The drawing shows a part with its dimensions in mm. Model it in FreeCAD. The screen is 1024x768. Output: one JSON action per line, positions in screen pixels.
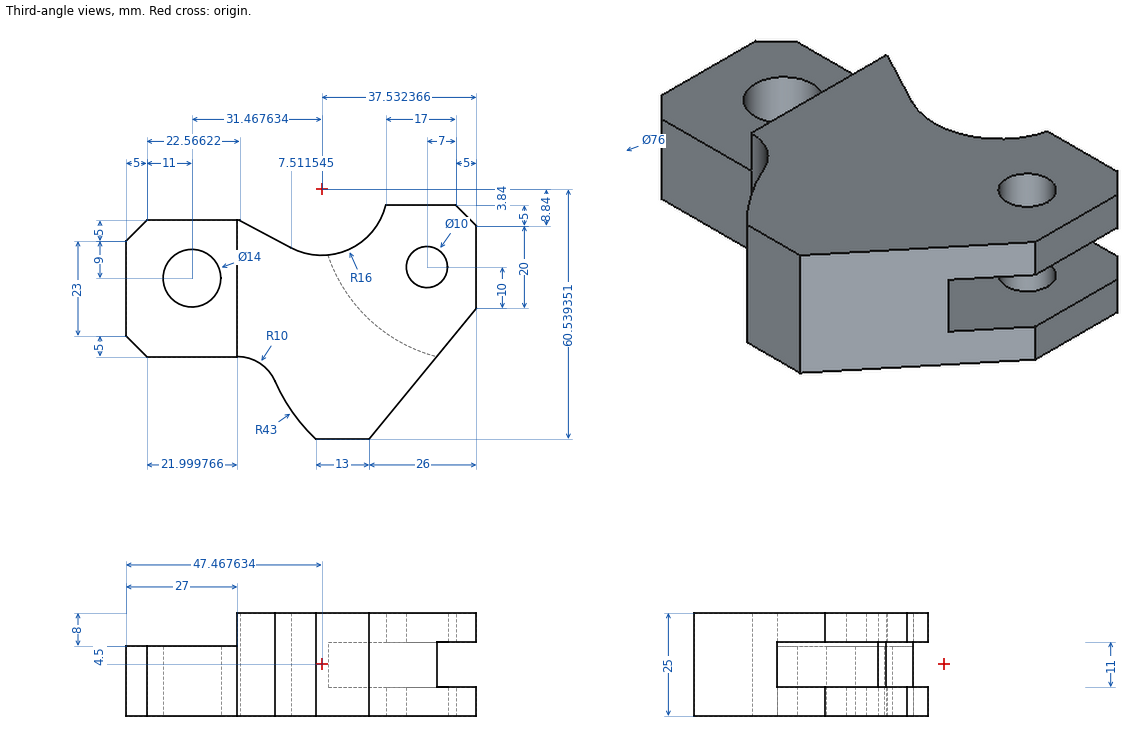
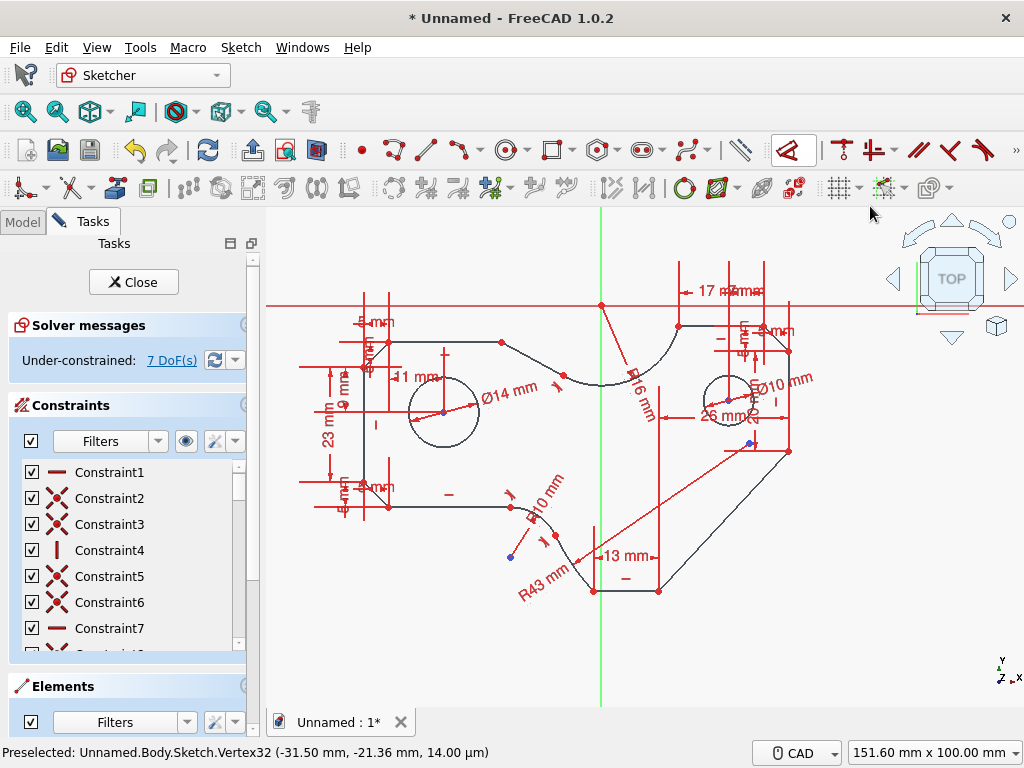
{"action": "left_click", "coordinate": [789, 451]}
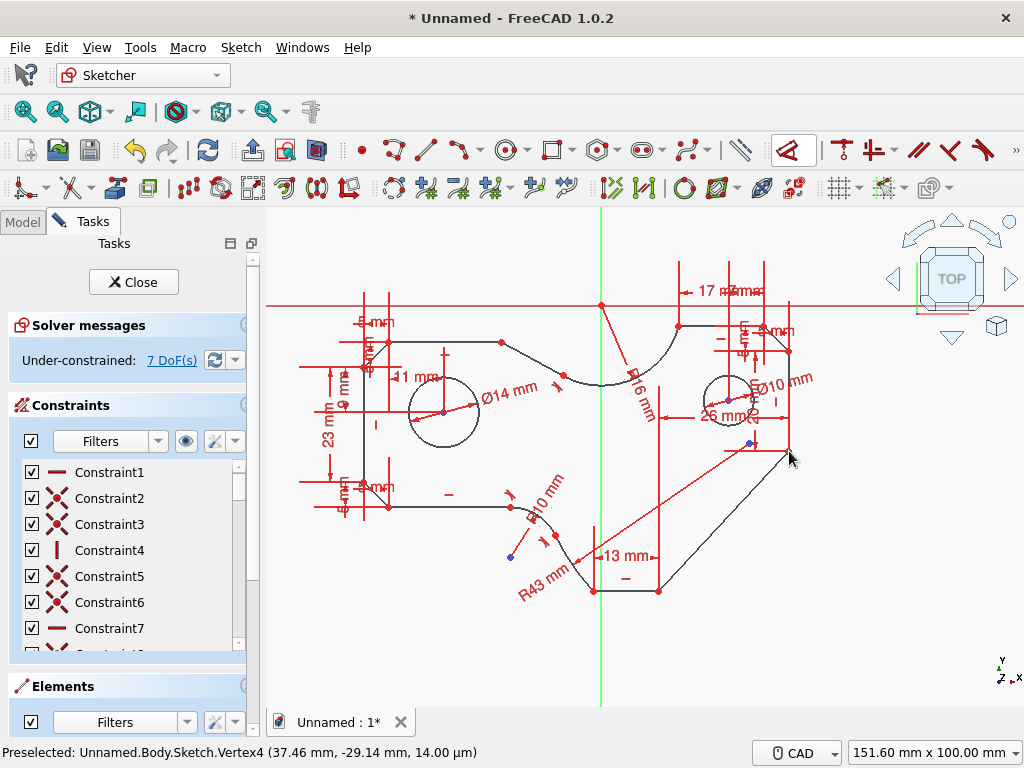
{"action": "left_click", "coordinate": [729, 401]}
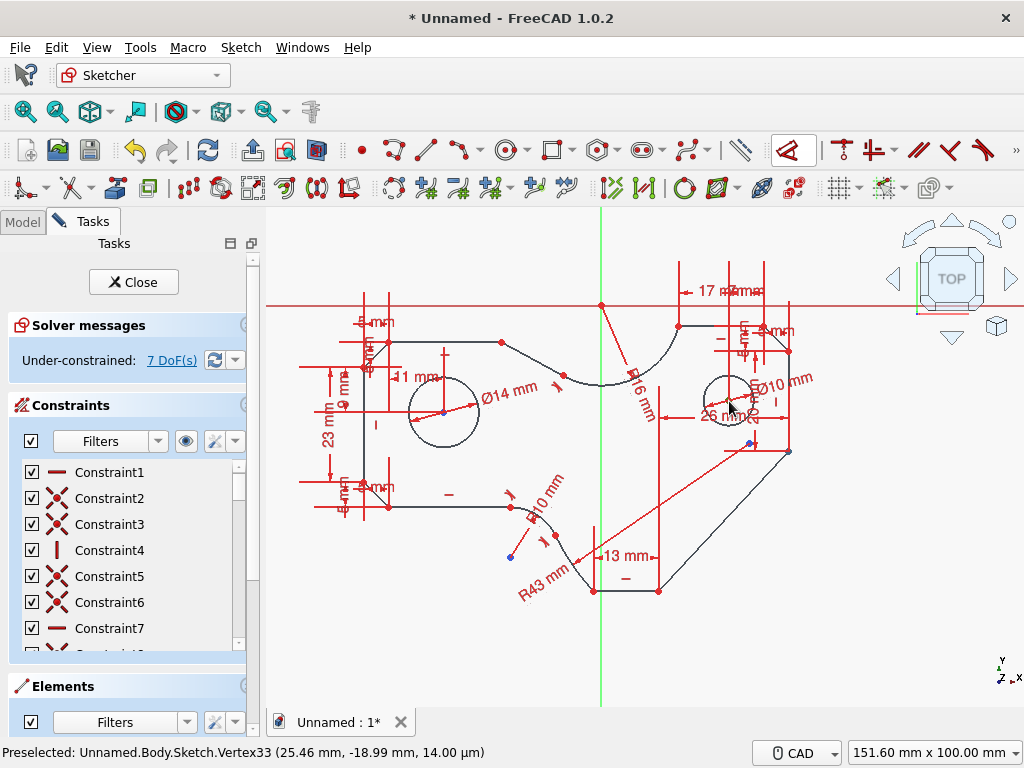
{"action": "left_click", "coordinate": [810, 150]}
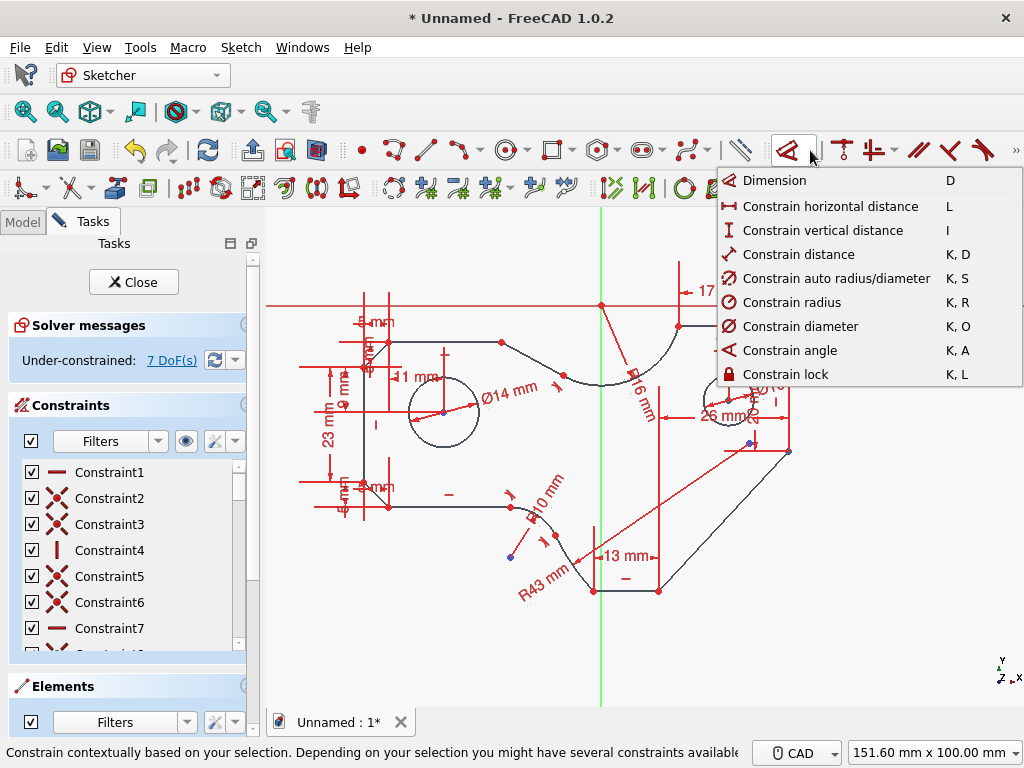
{"action": "left_click", "coordinate": [870, 230]}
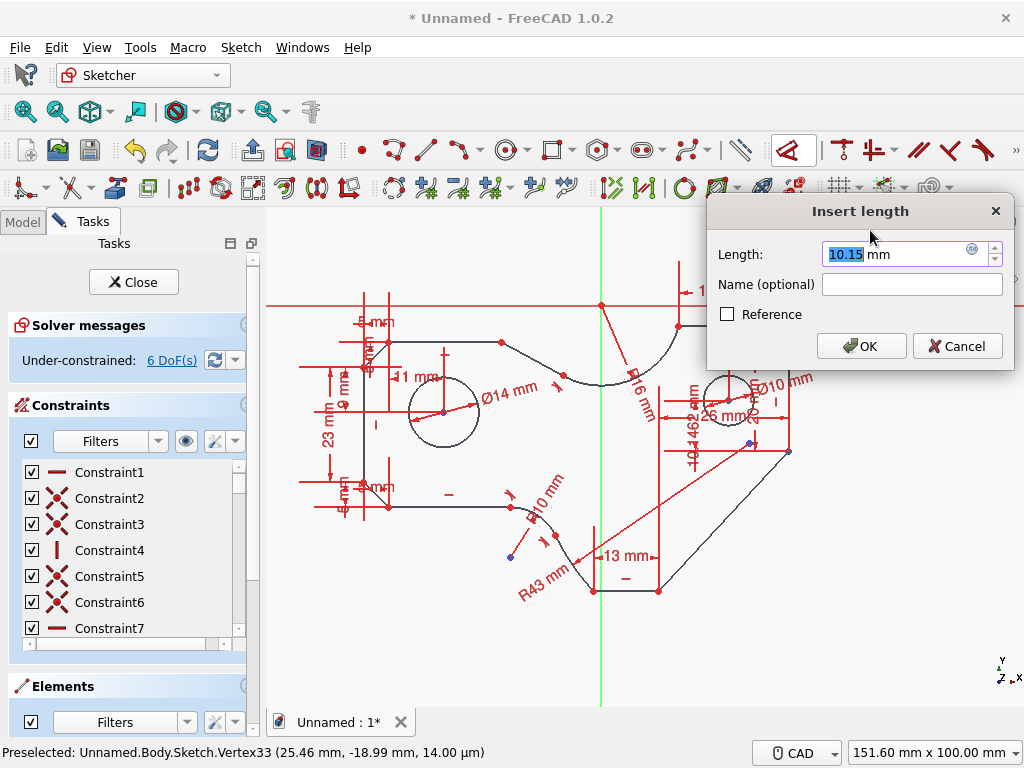
{"action": "type", "text": "10"}
{"action": "key", "text": "Return"}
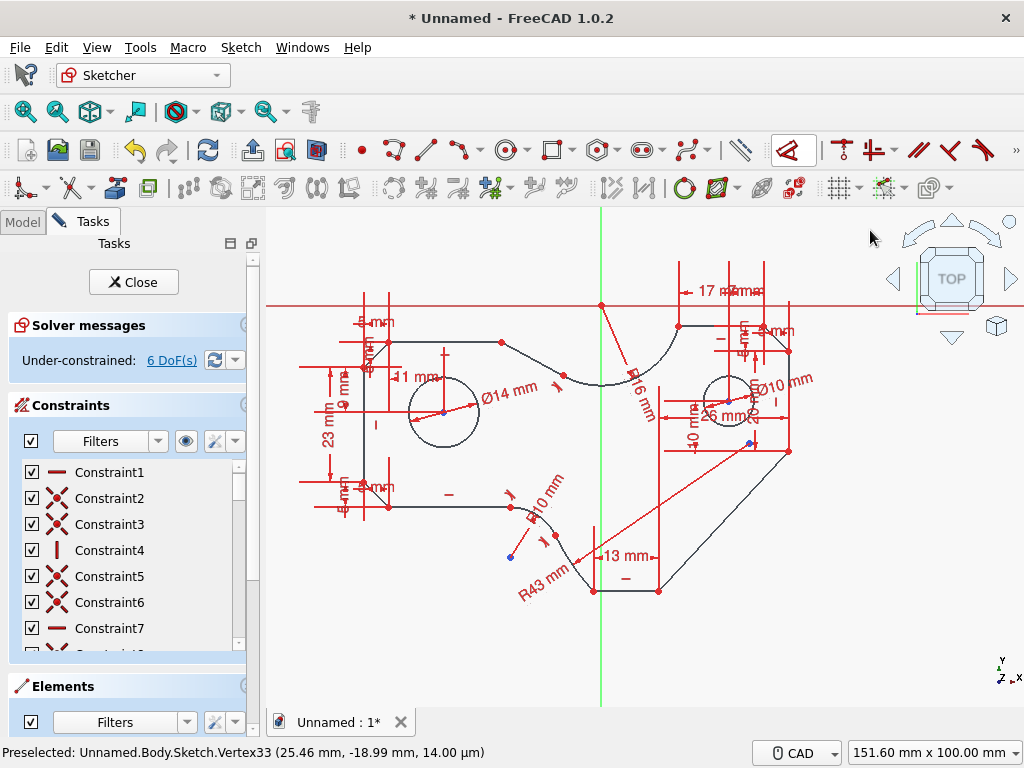
{"action": "left_click", "coordinate": [789, 351]}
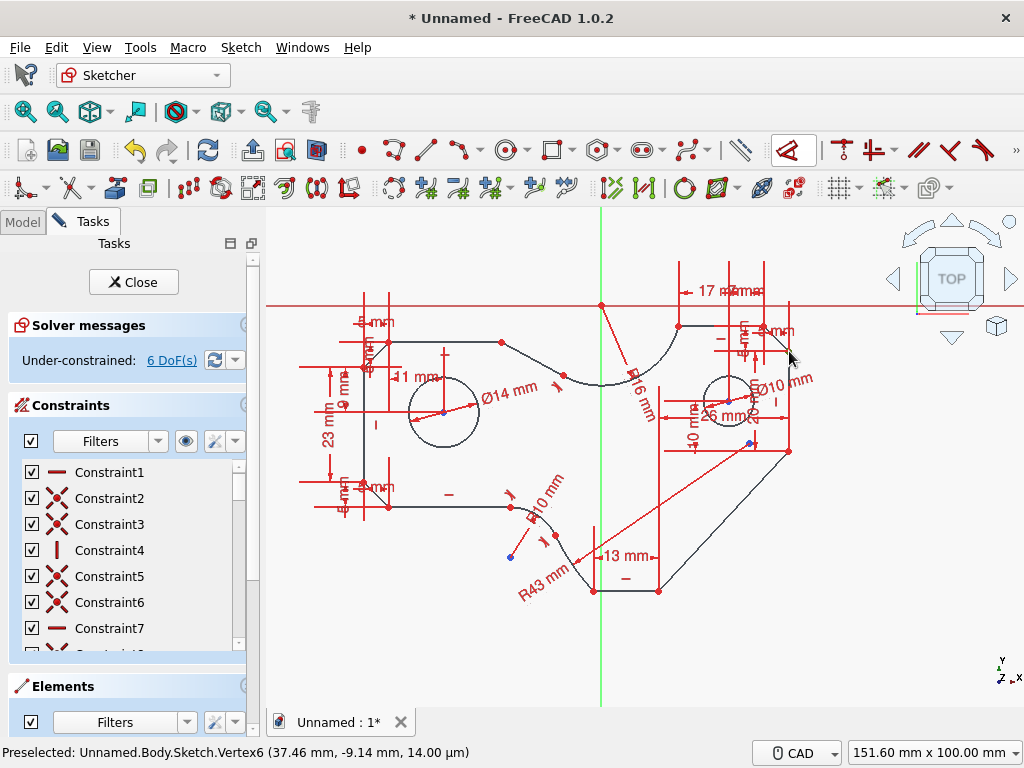
{"action": "left_click", "coordinate": [810, 150]}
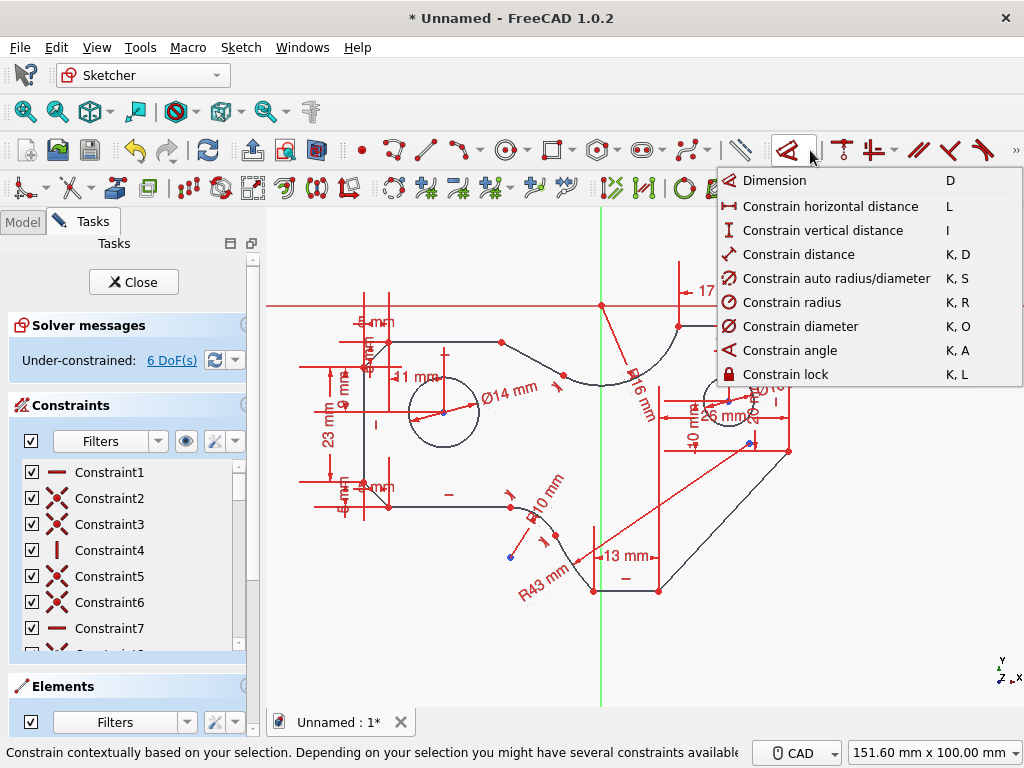
{"action": "left_click", "coordinate": [870, 230]}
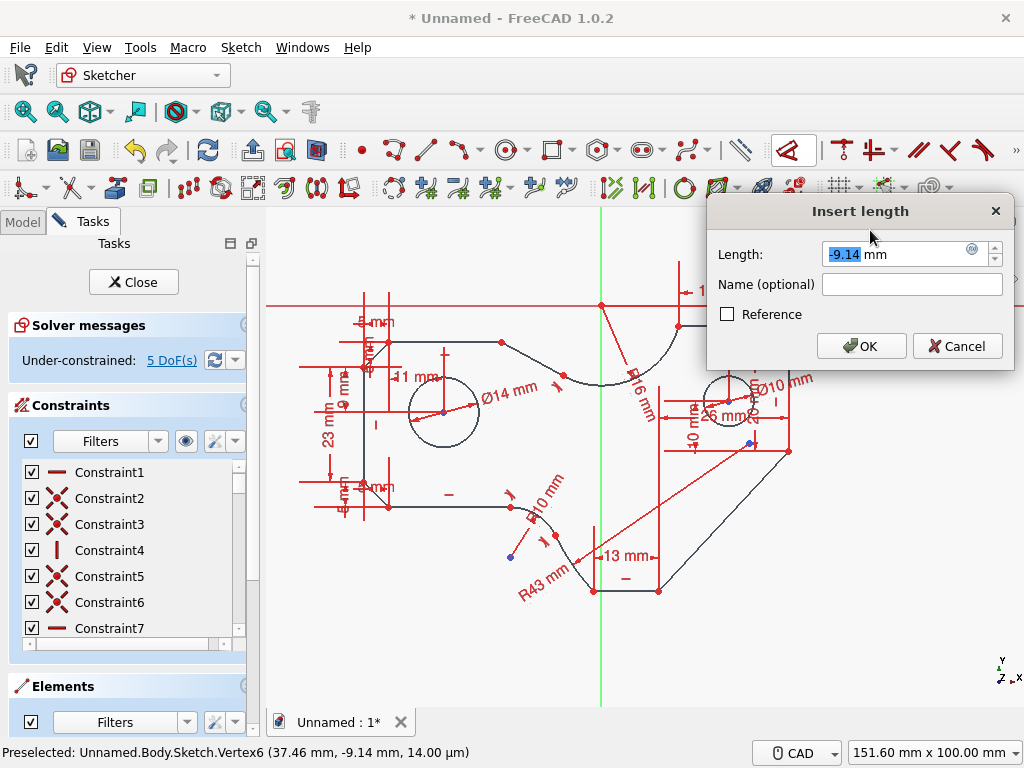
{"action": "type", "text": "-8.84"}
{"action": "key", "text": "Return"}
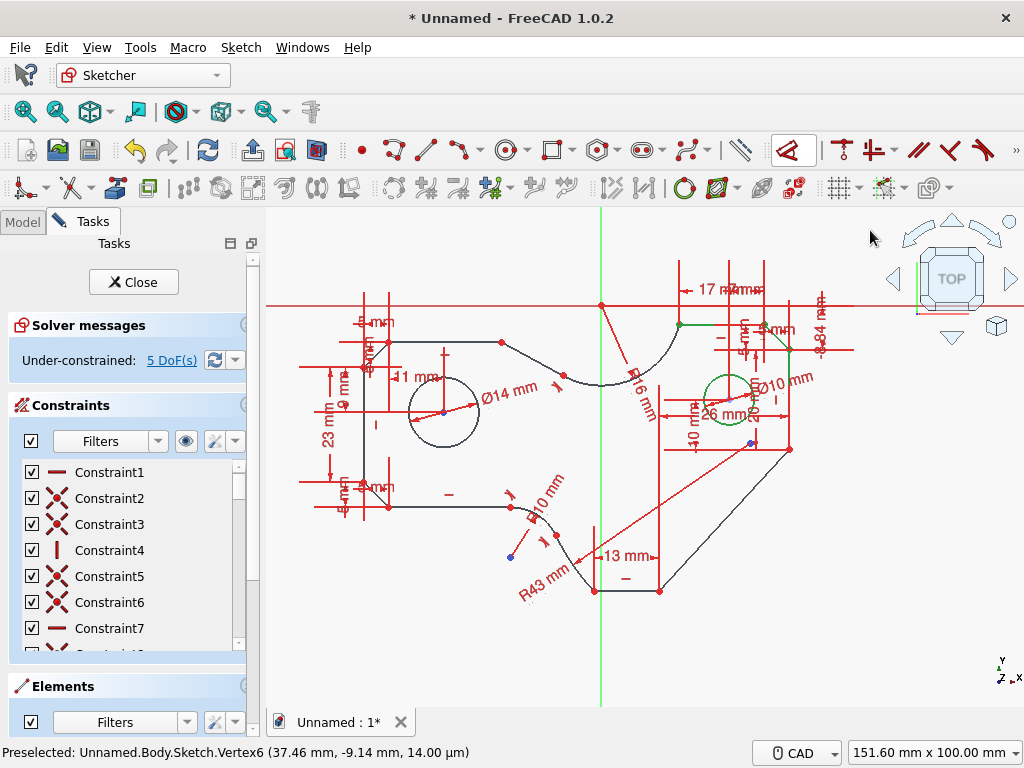
{"action": "left_click", "coordinate": [468, 342]}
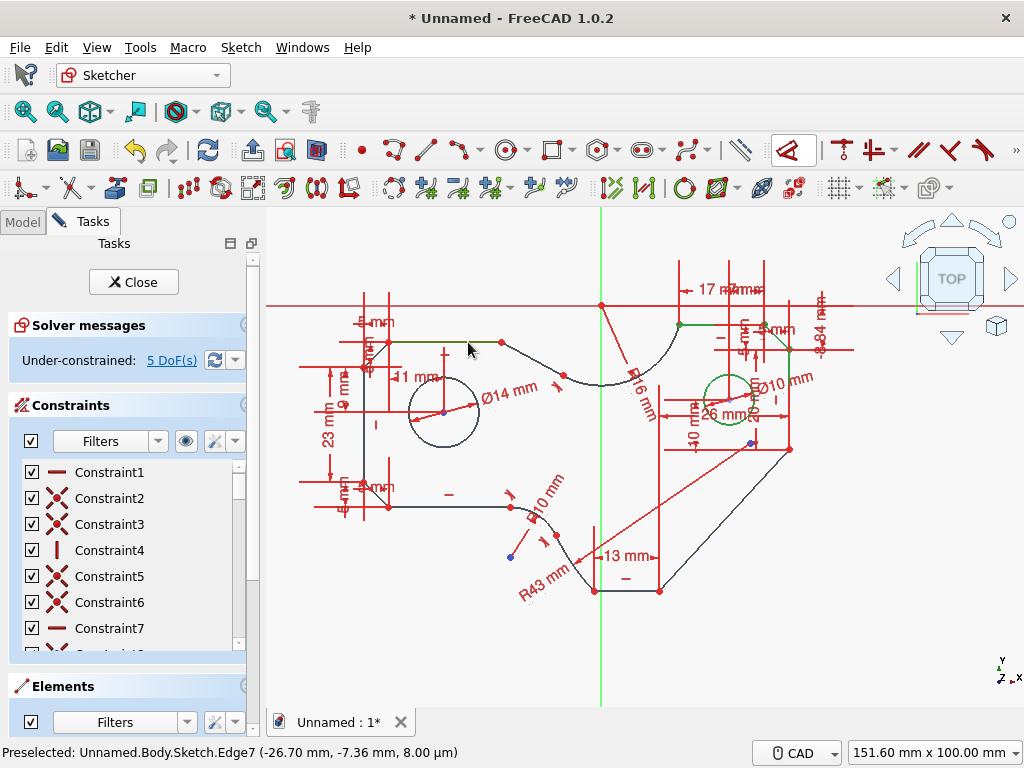
{"action": "key", "text": "l"}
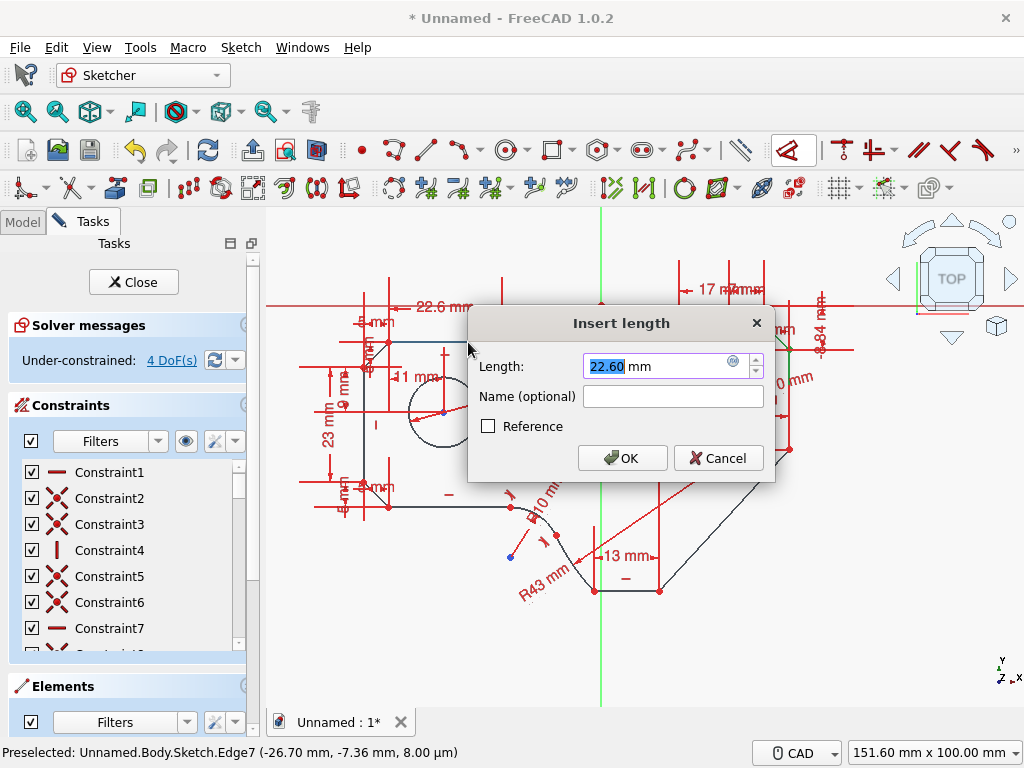
{"action": "type", "text": "22.56622"}
{"action": "key", "text": "Return"}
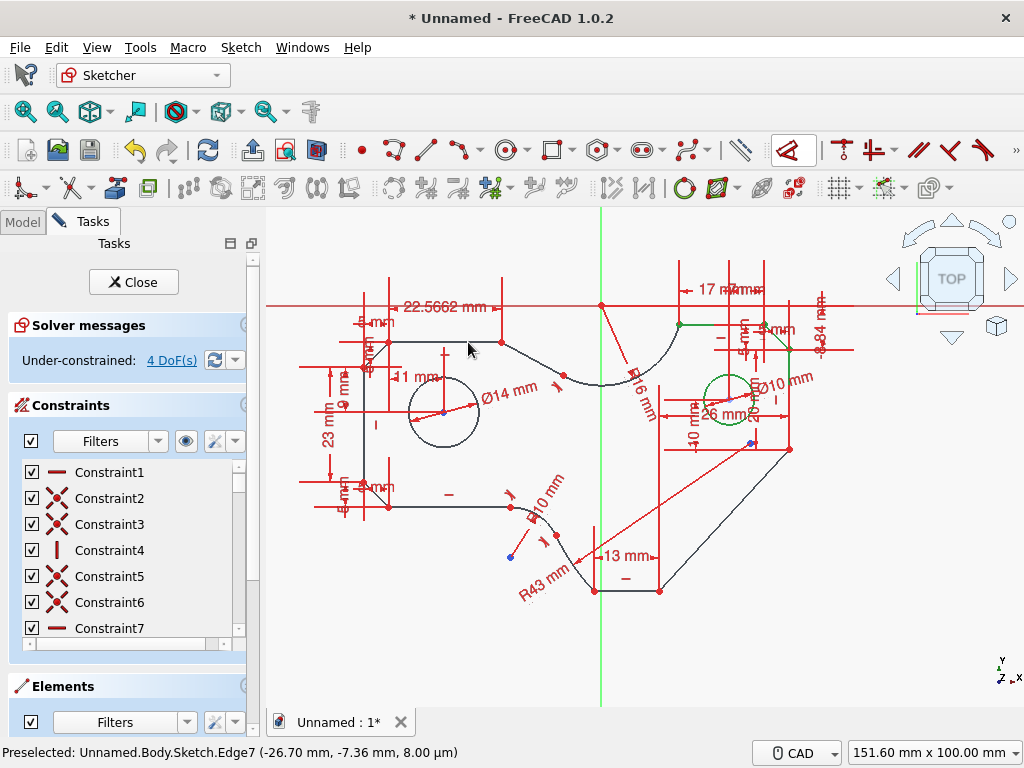
{"action": "left_click", "coordinate": [425, 507]}